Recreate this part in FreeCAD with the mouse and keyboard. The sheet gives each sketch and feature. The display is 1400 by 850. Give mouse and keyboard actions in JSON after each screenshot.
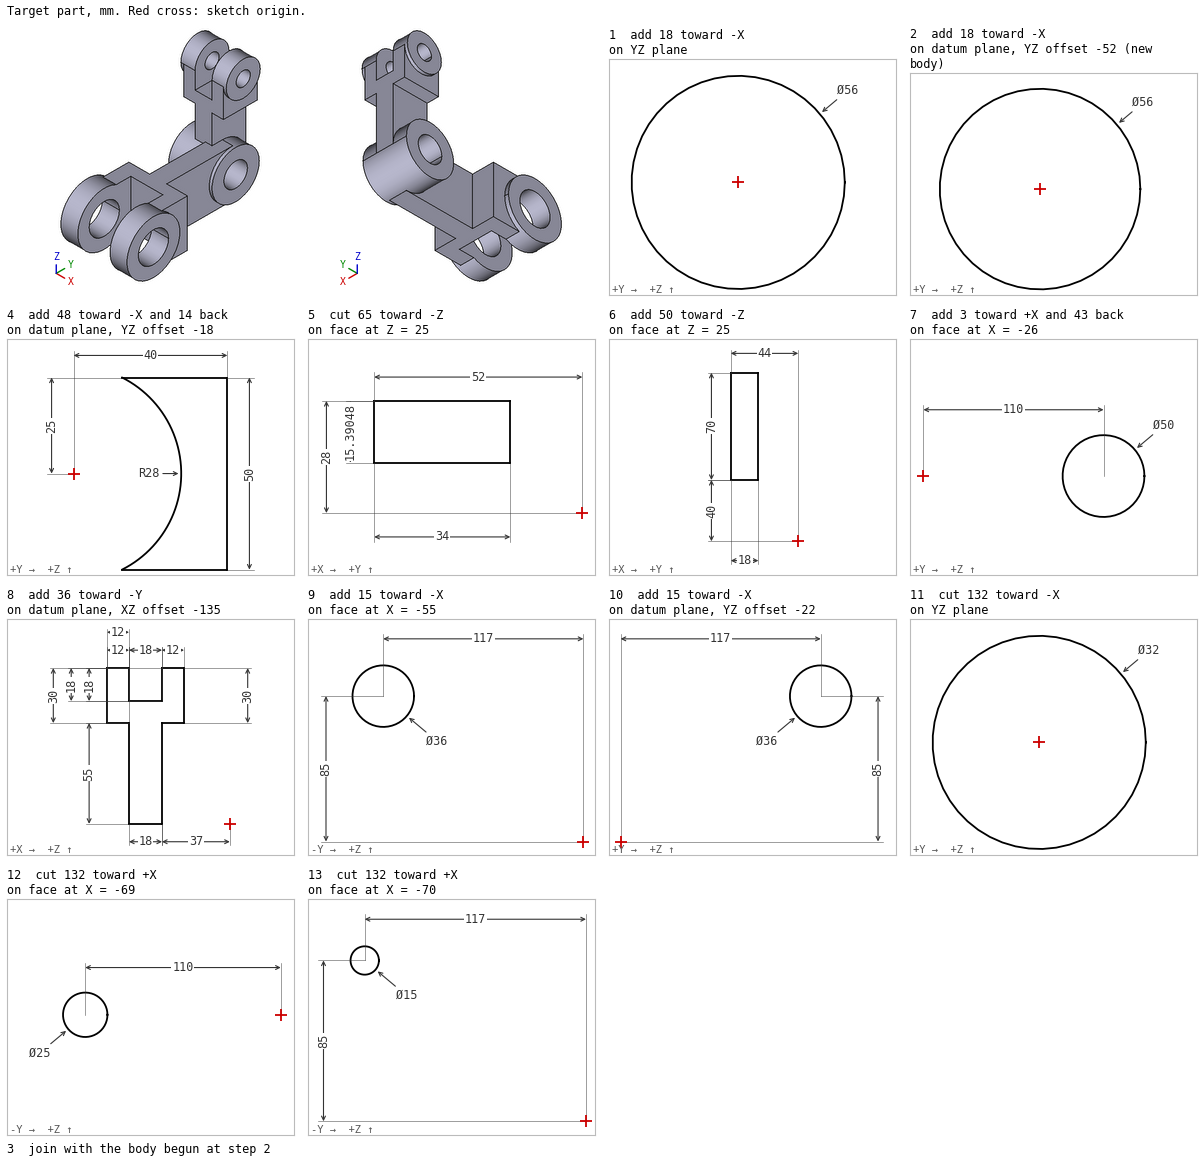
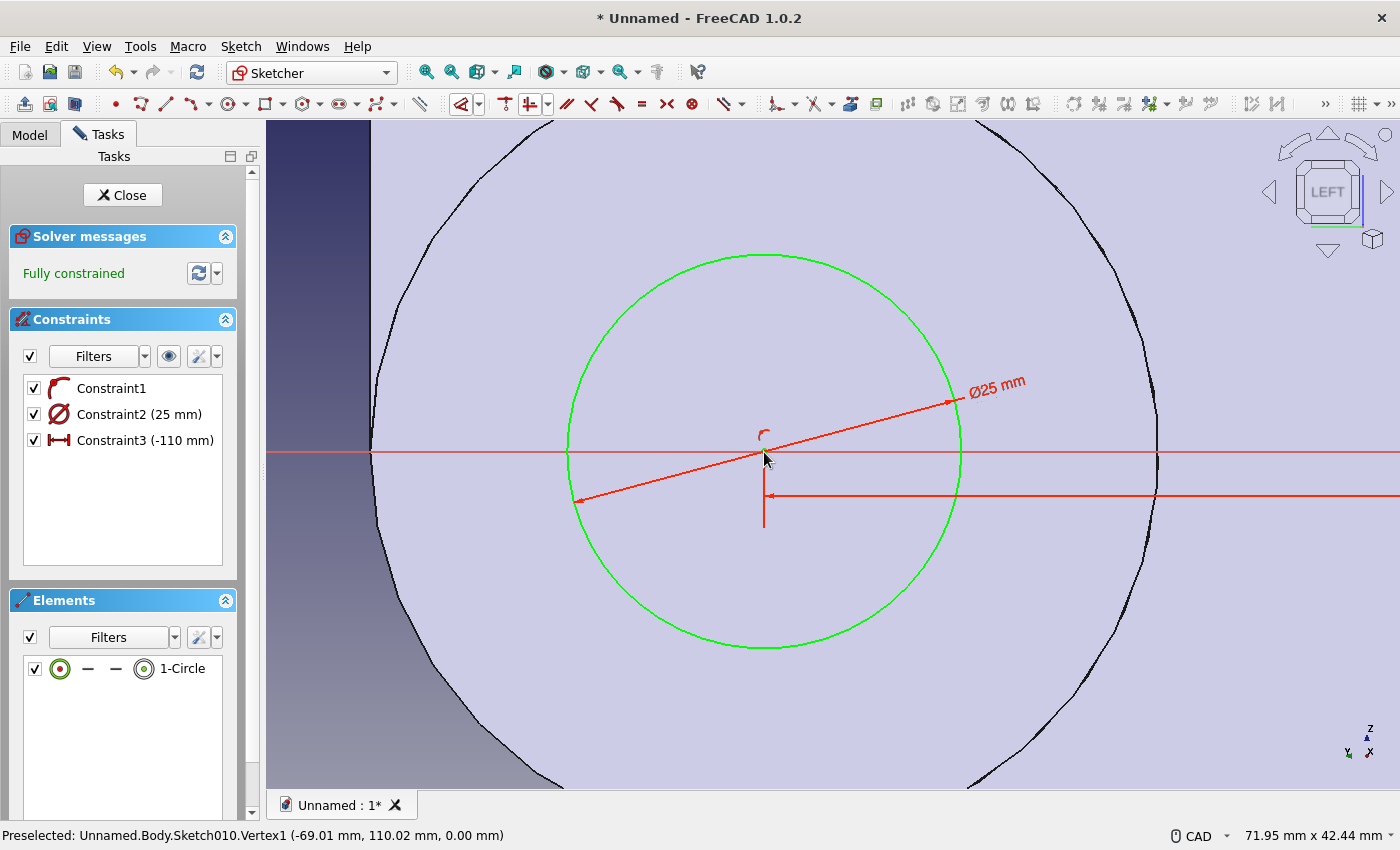
{"action": "left_click", "coordinate": [123, 195]}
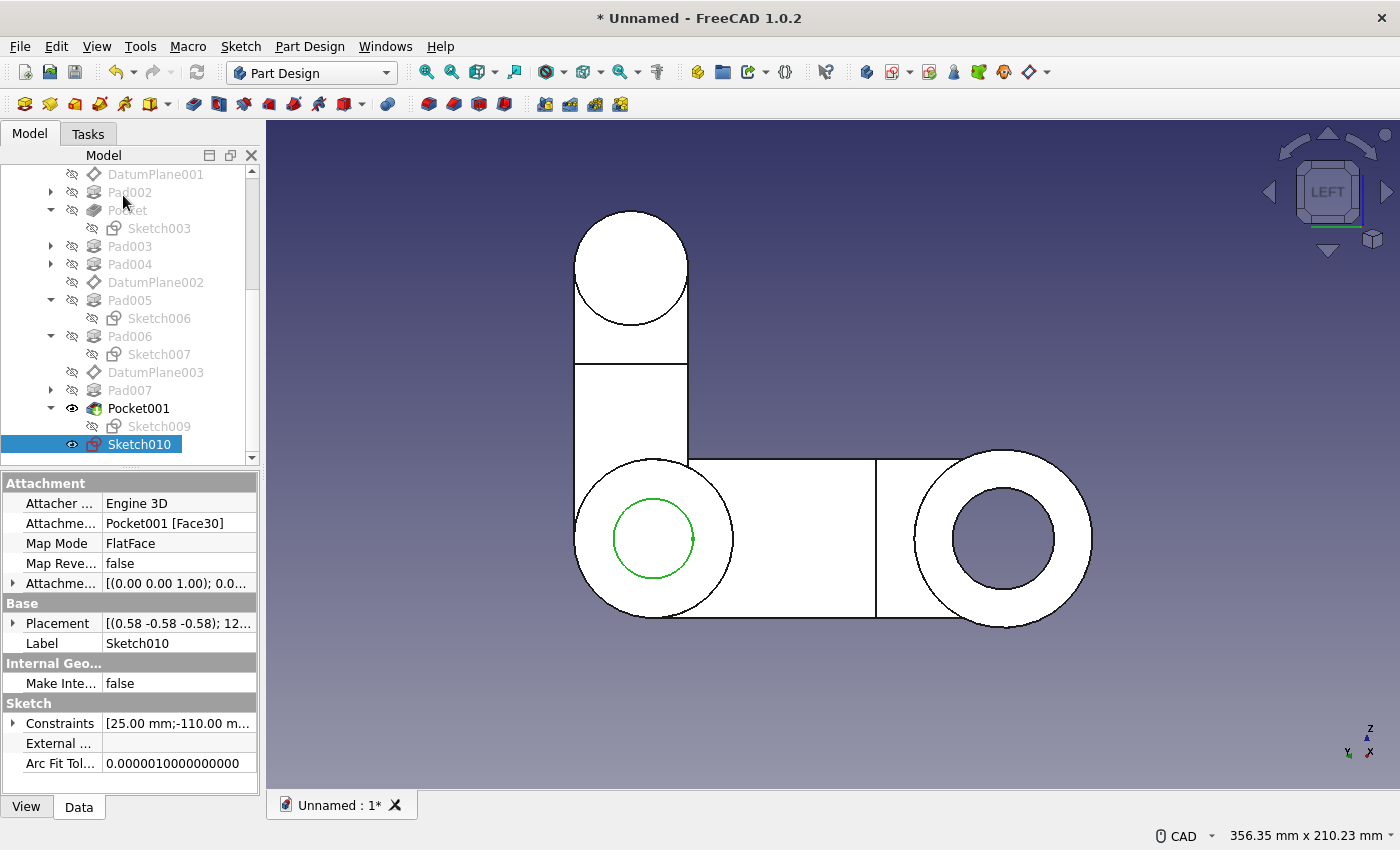
{"action": "left_click", "coordinate": [194, 104]}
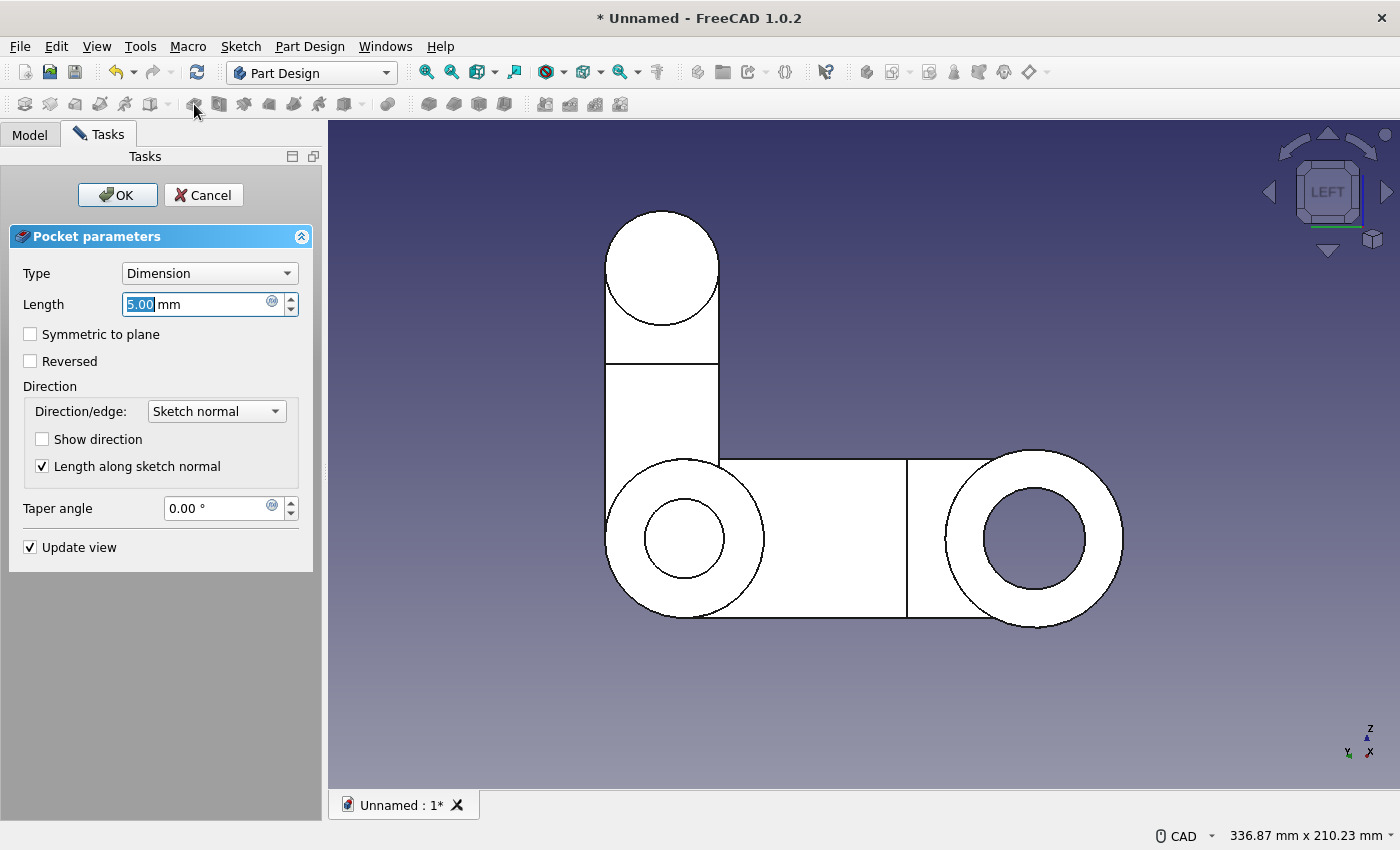
{"action": "type", "text": "132"}
{"action": "key", "text": "Tab"}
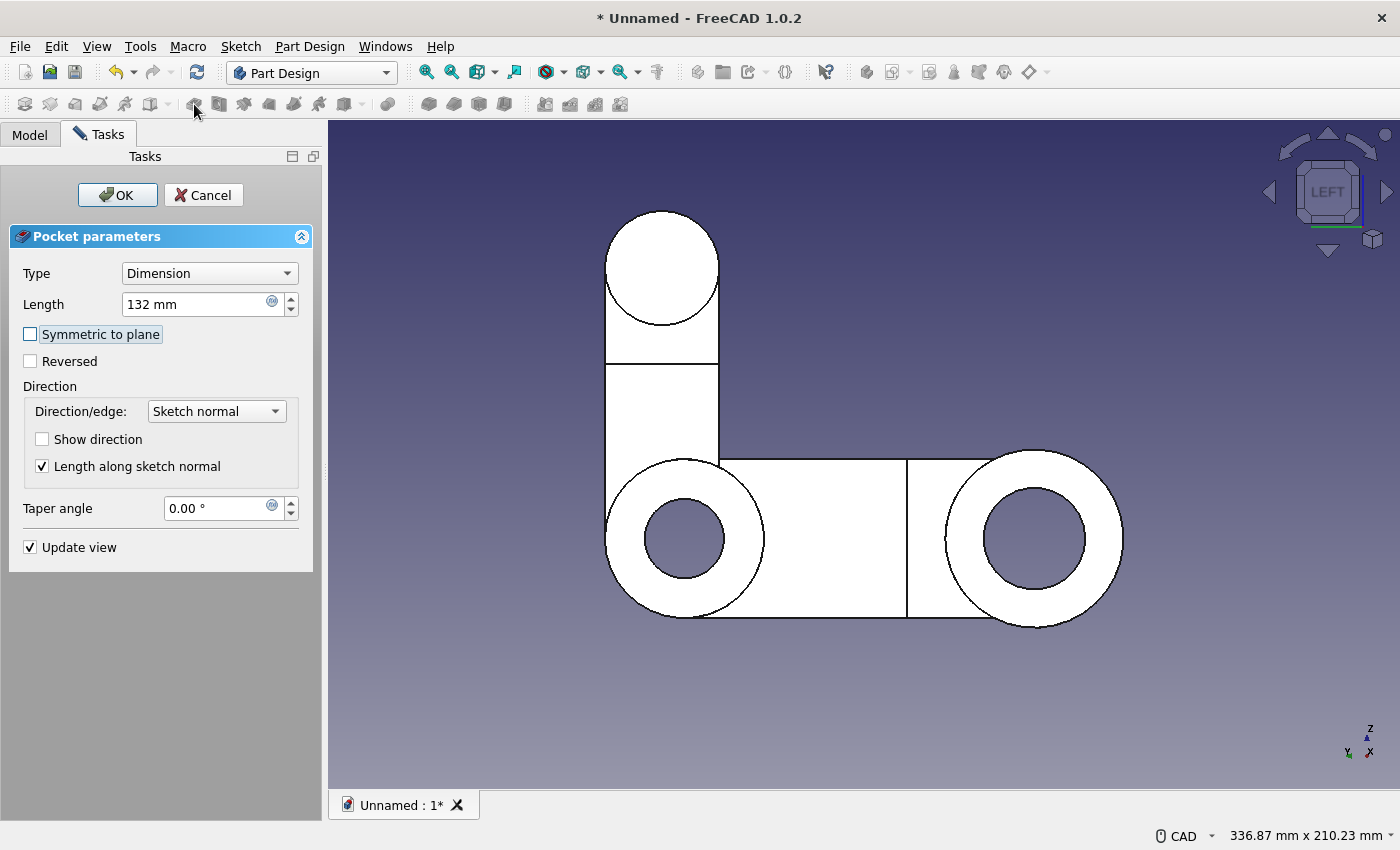
{"action": "left_click", "coordinate": [118, 195]}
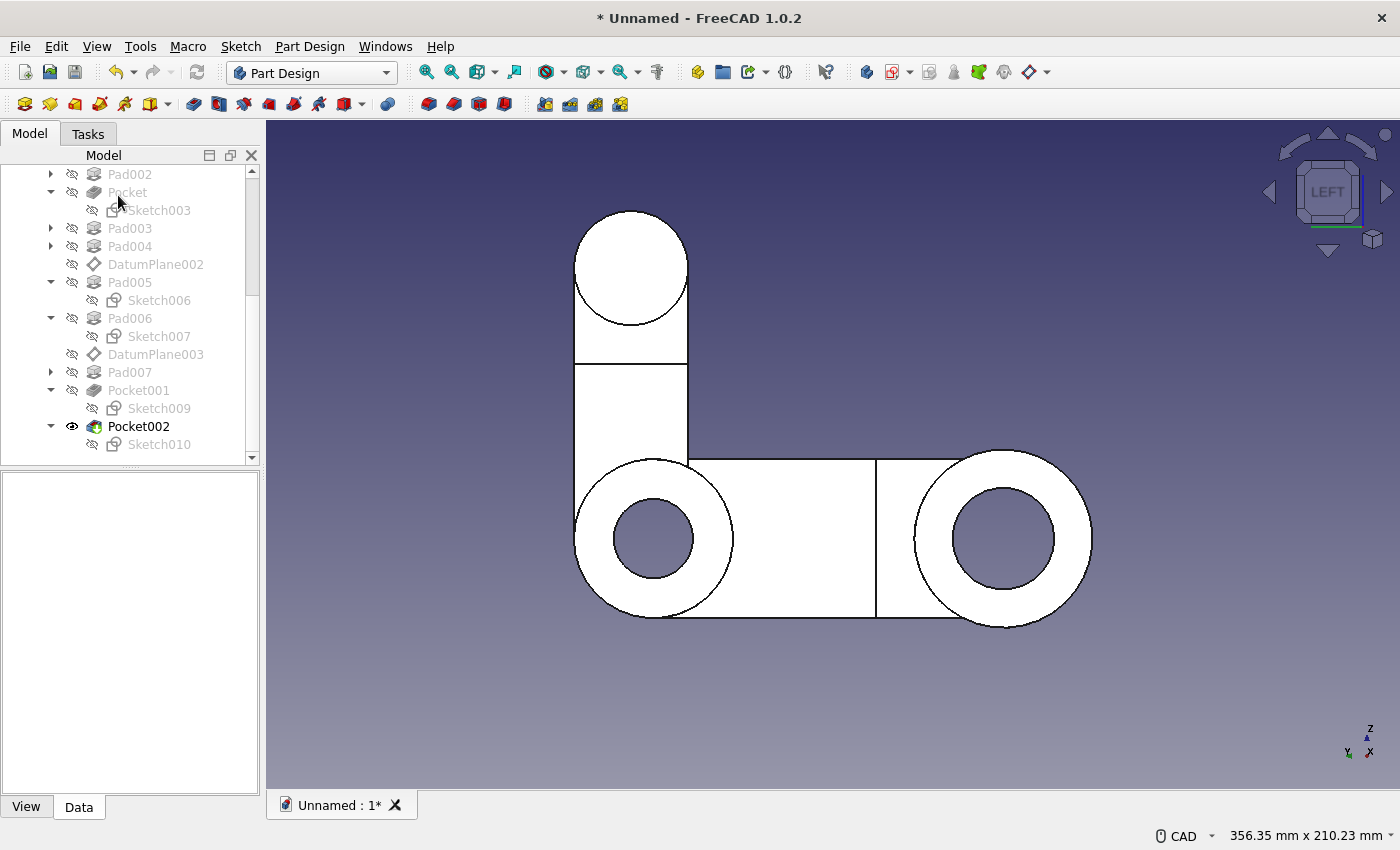
{"action": "left_click", "coordinate": [953, 487]}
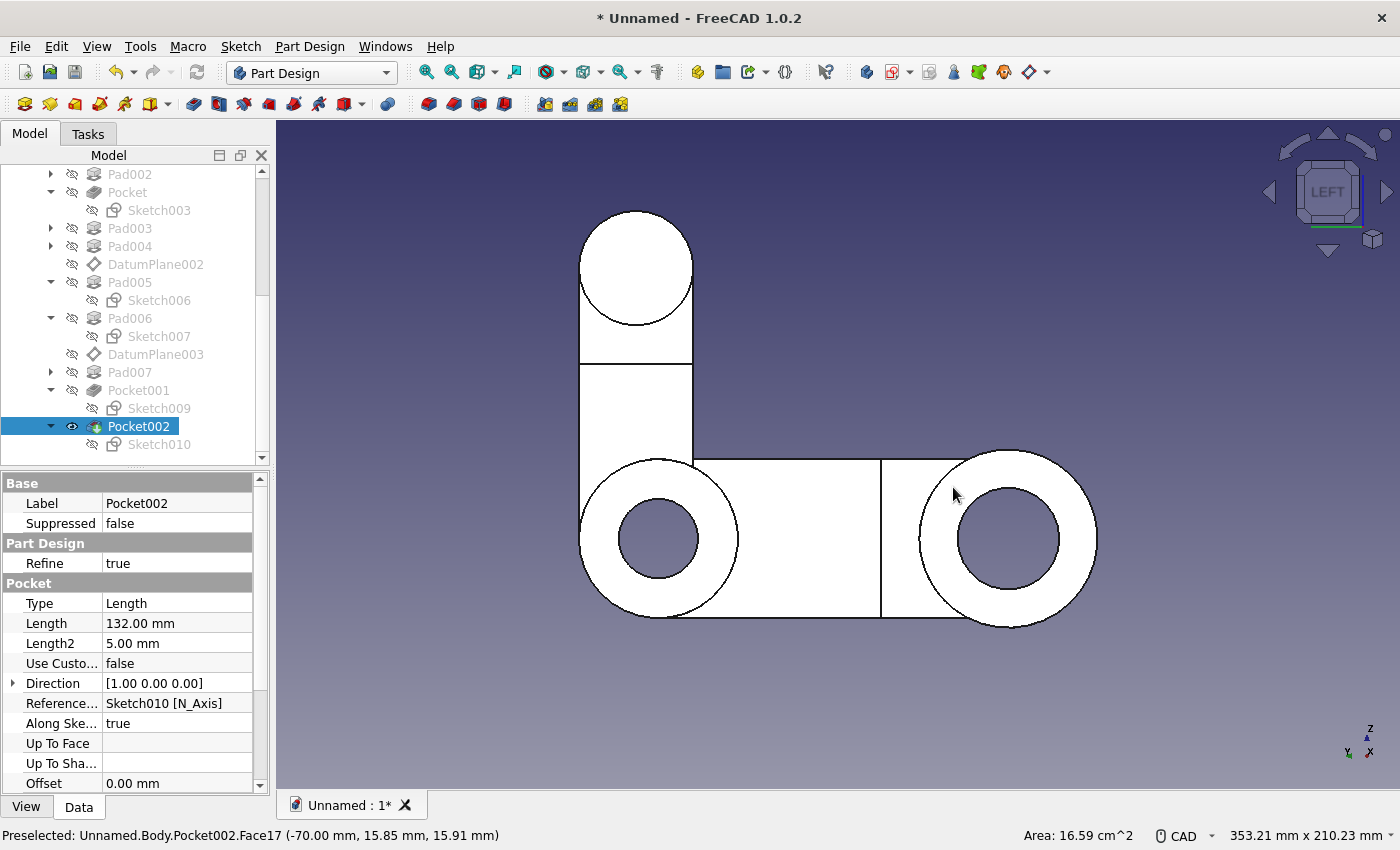
{"action": "left_click", "coordinate": [892, 72]}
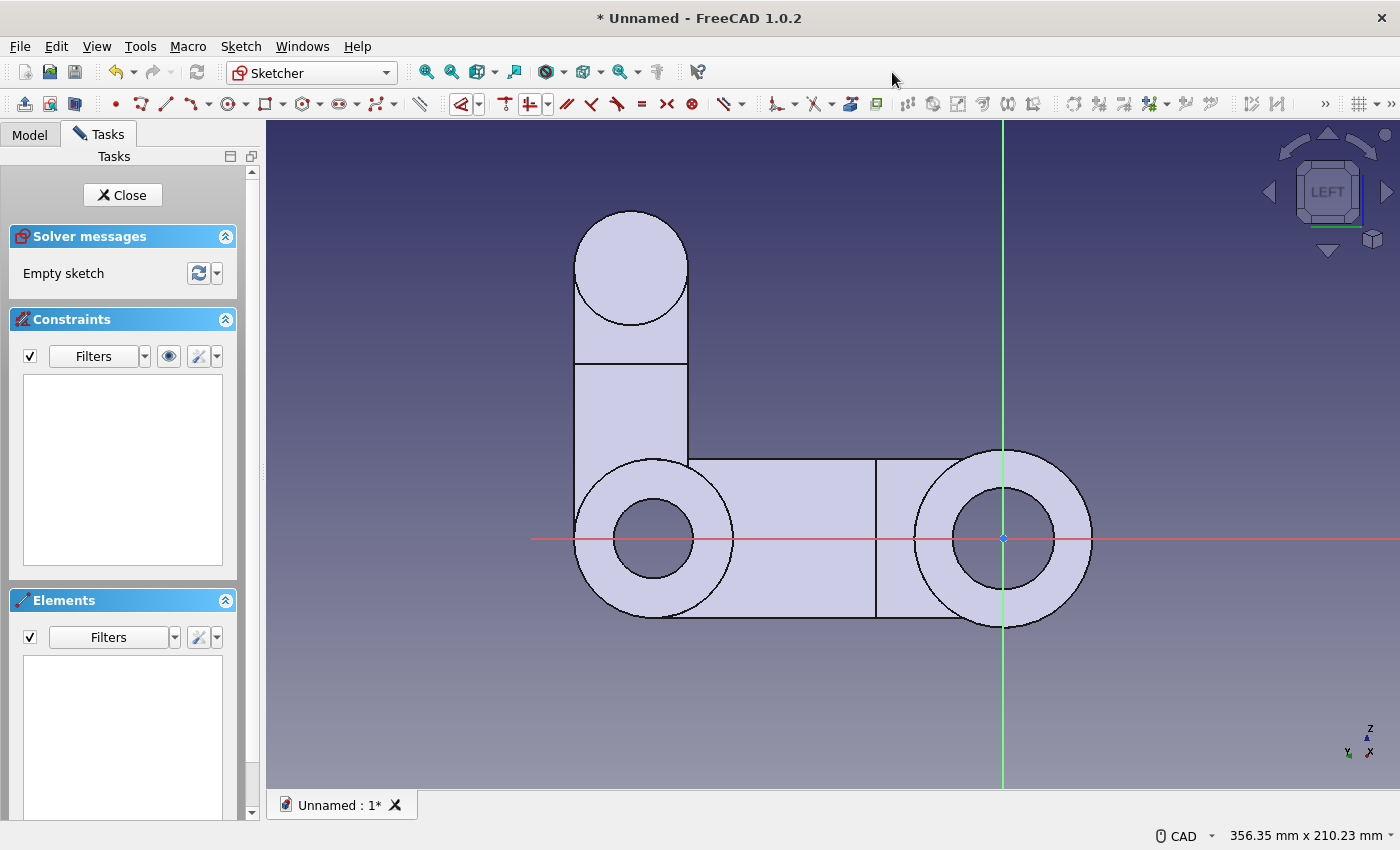
{"action": "scroll", "coordinate": [614, 245], "scroll_direction": "up", "scroll_amount": 11}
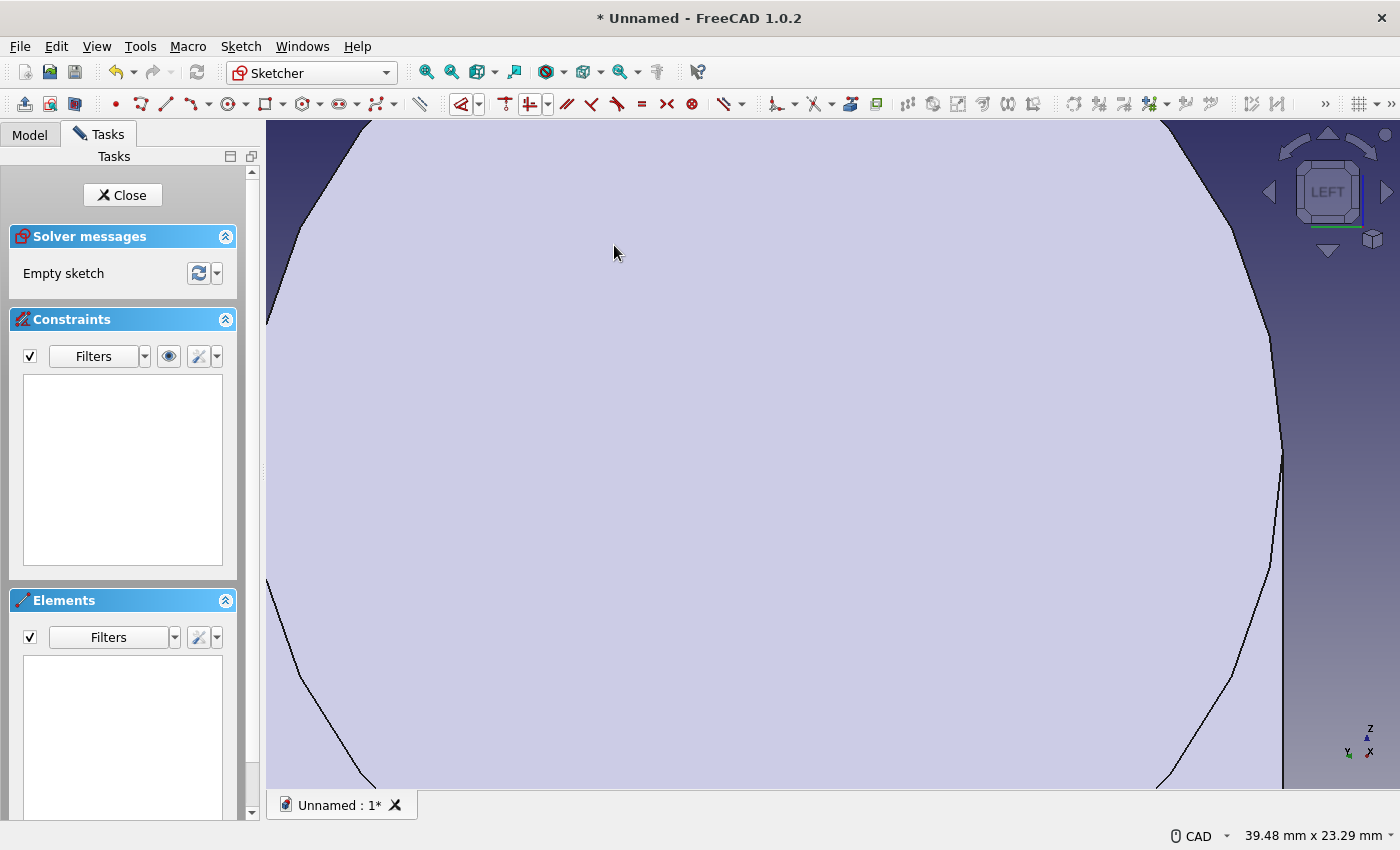
{"action": "key", "text": "g c"}